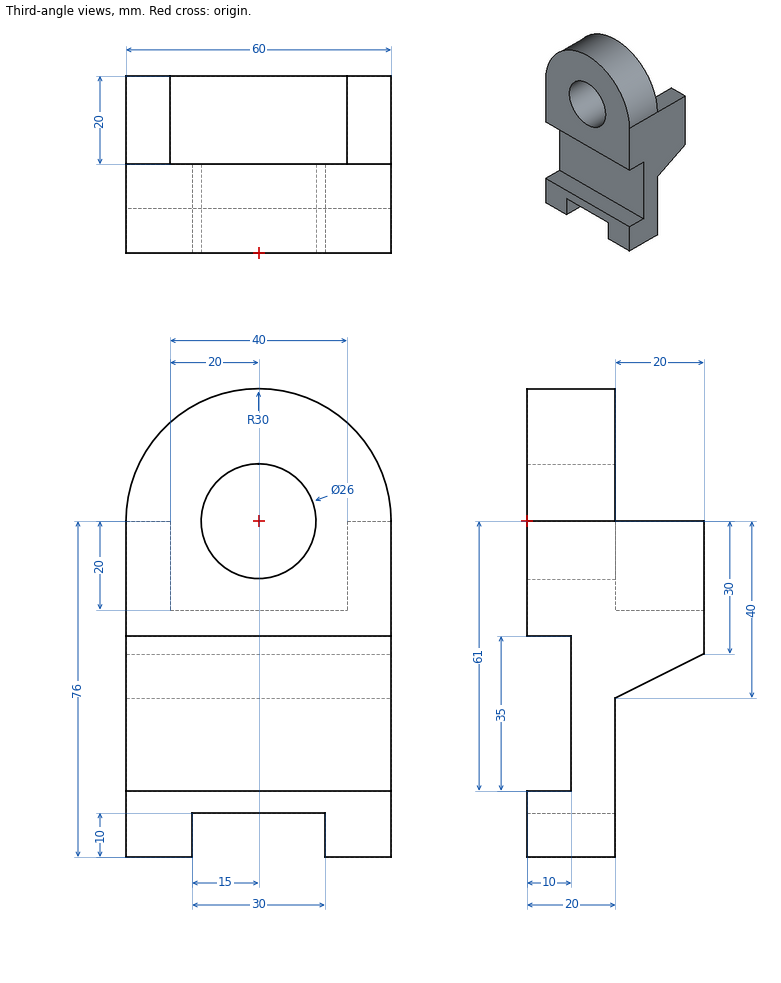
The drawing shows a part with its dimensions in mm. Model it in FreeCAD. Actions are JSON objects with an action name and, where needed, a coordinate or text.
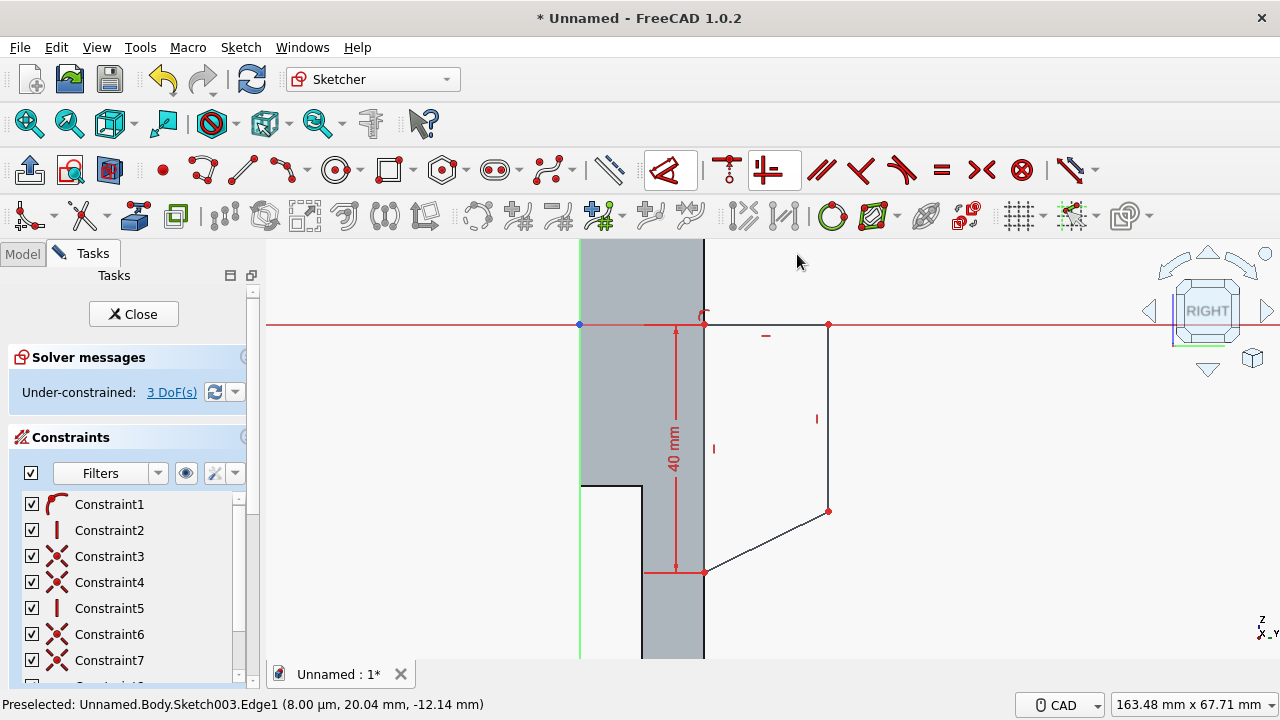
{"action": "left_click", "coordinate": [828, 456]}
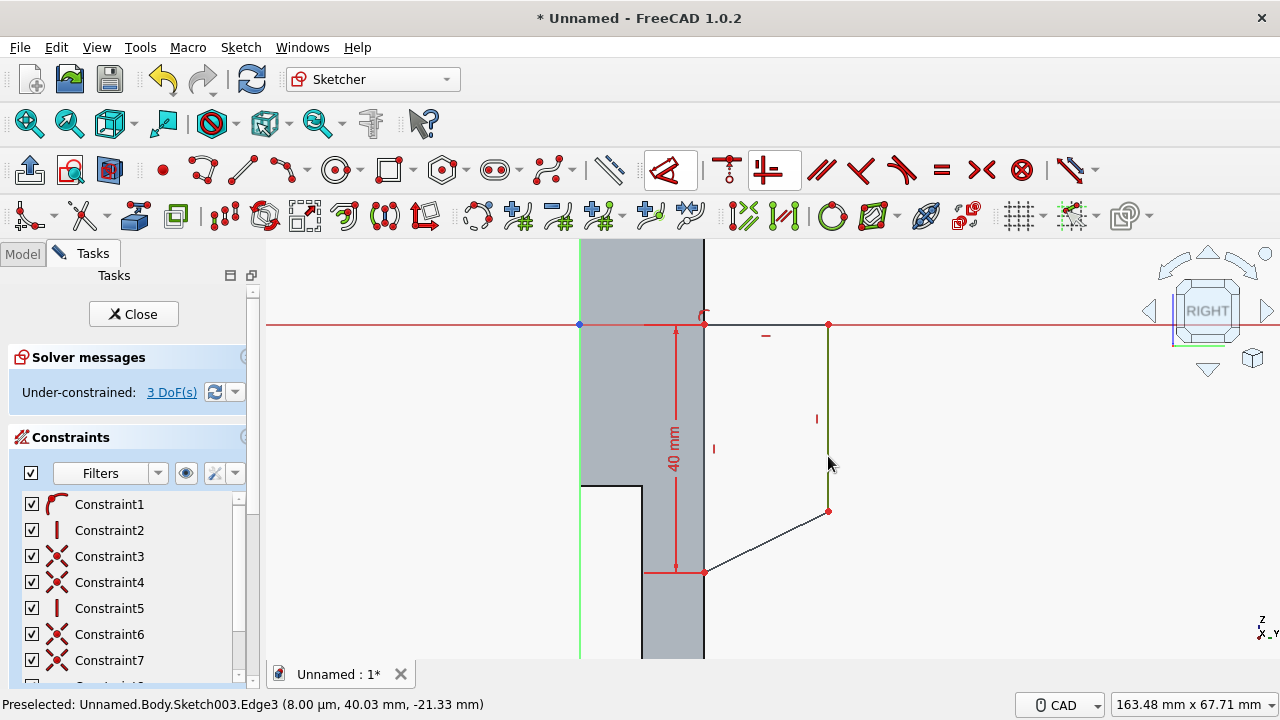
{"action": "key", "text": "i"}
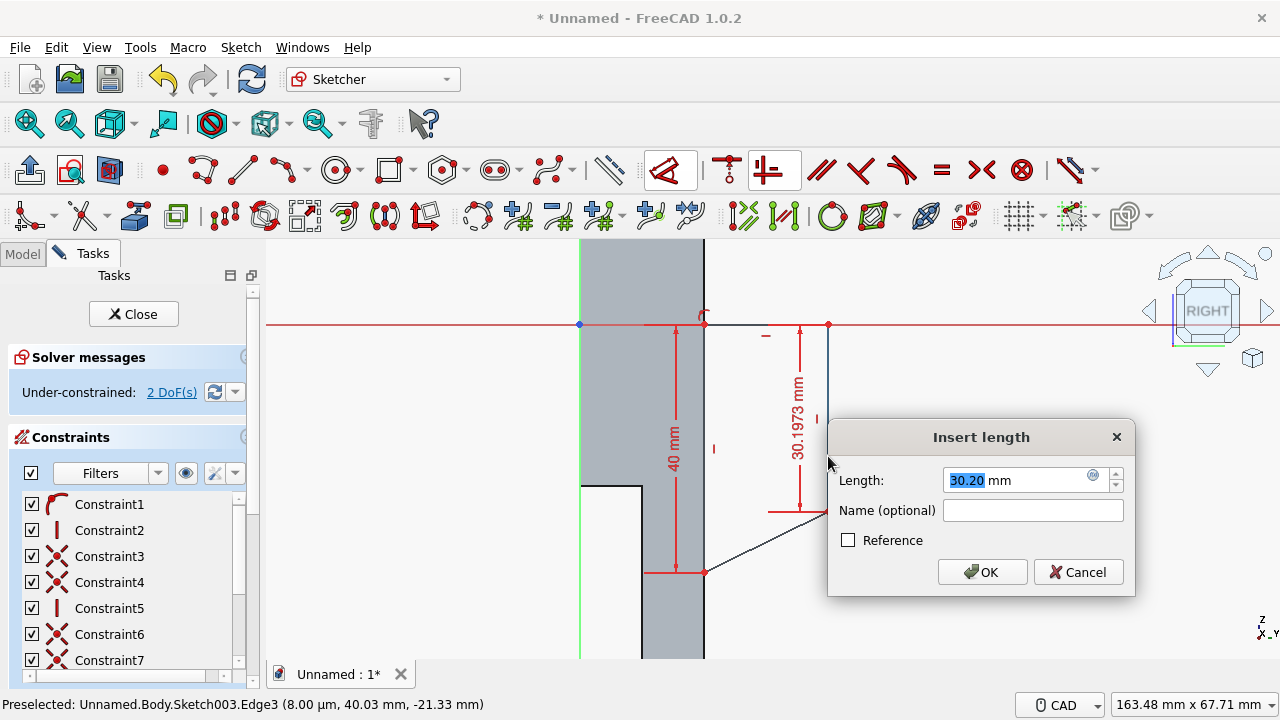
{"action": "type", "text": "30"}
{"action": "key", "text": "Return"}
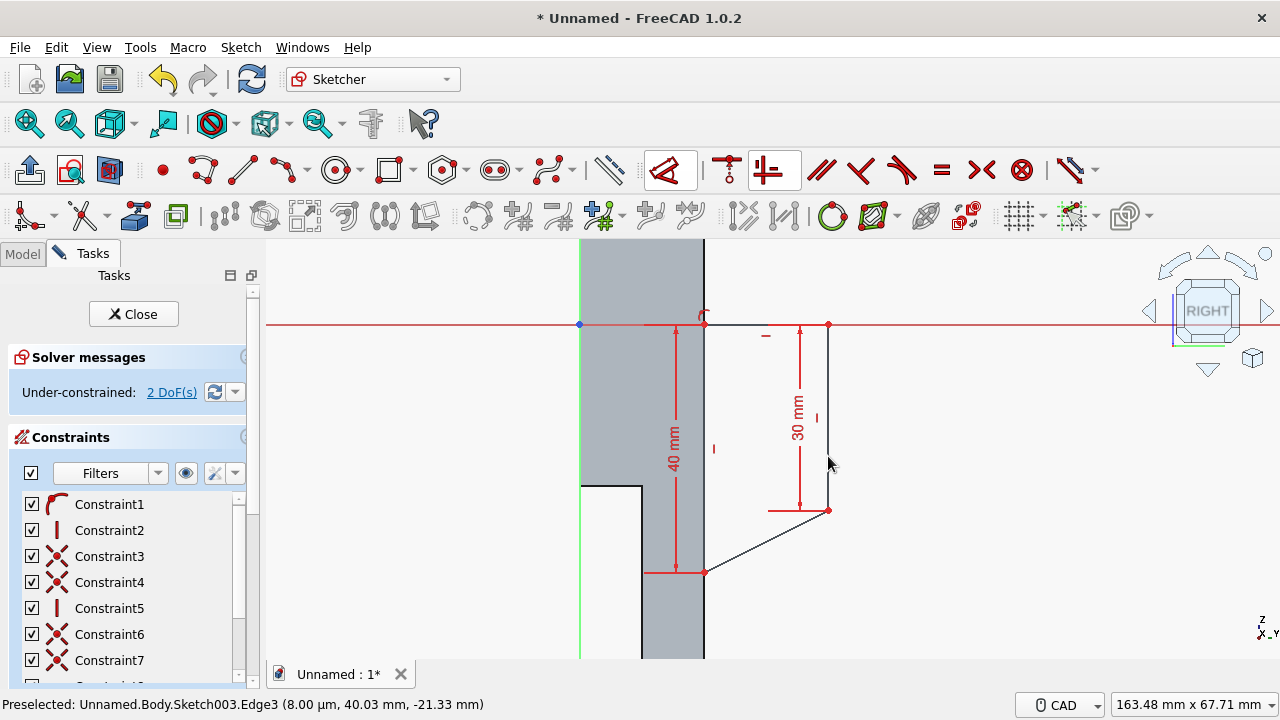
{"action": "left_click", "coordinate": [791, 325]}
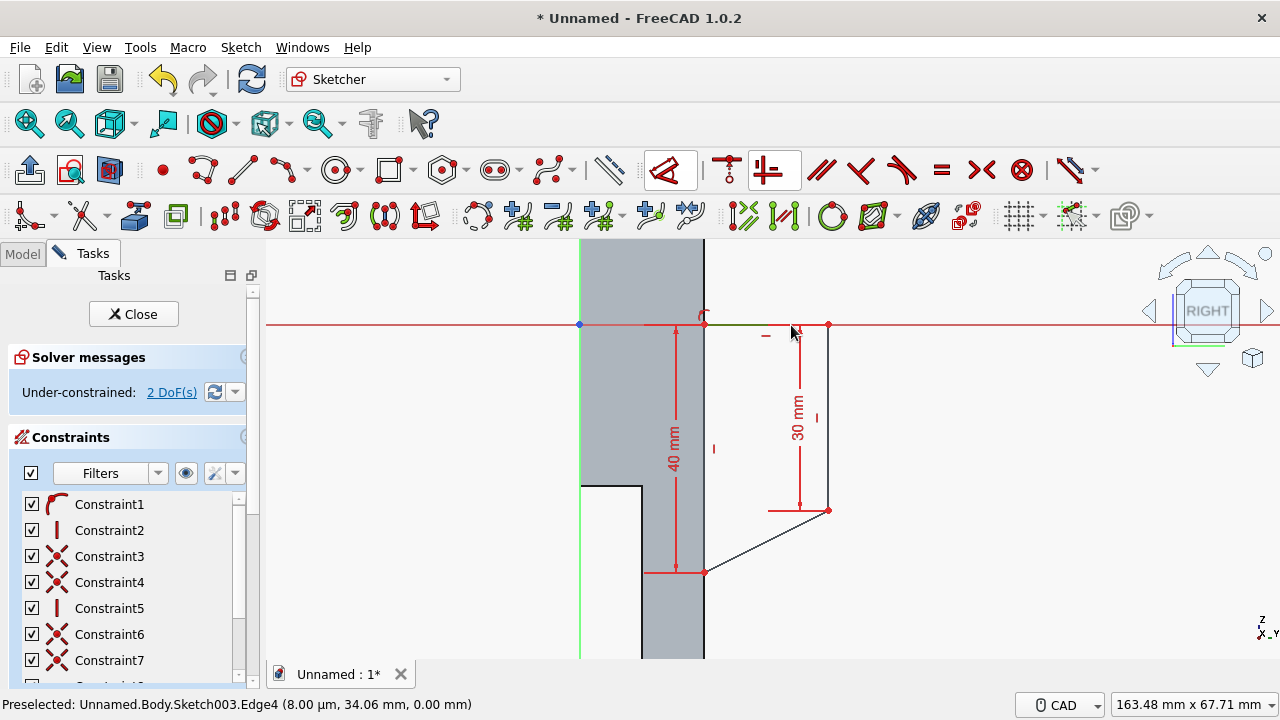
{"action": "left_click", "coordinate": [692, 170]}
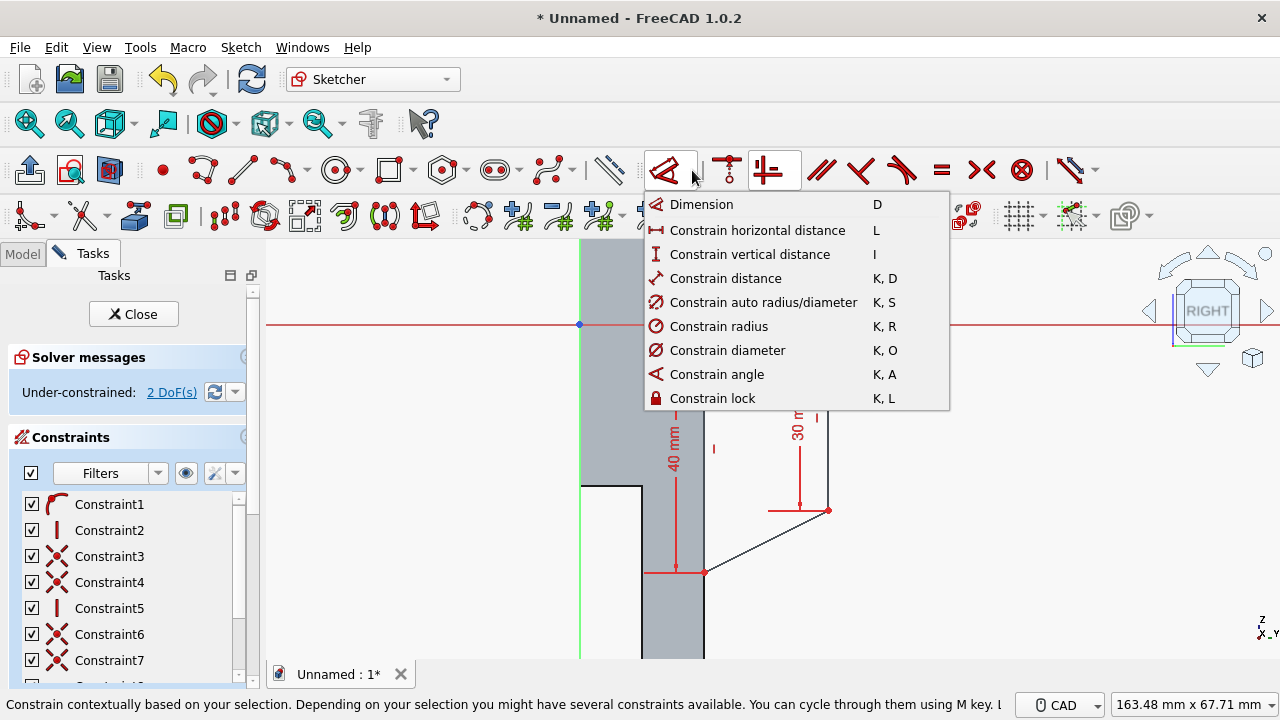
{"action": "left_click", "coordinate": [797, 230]}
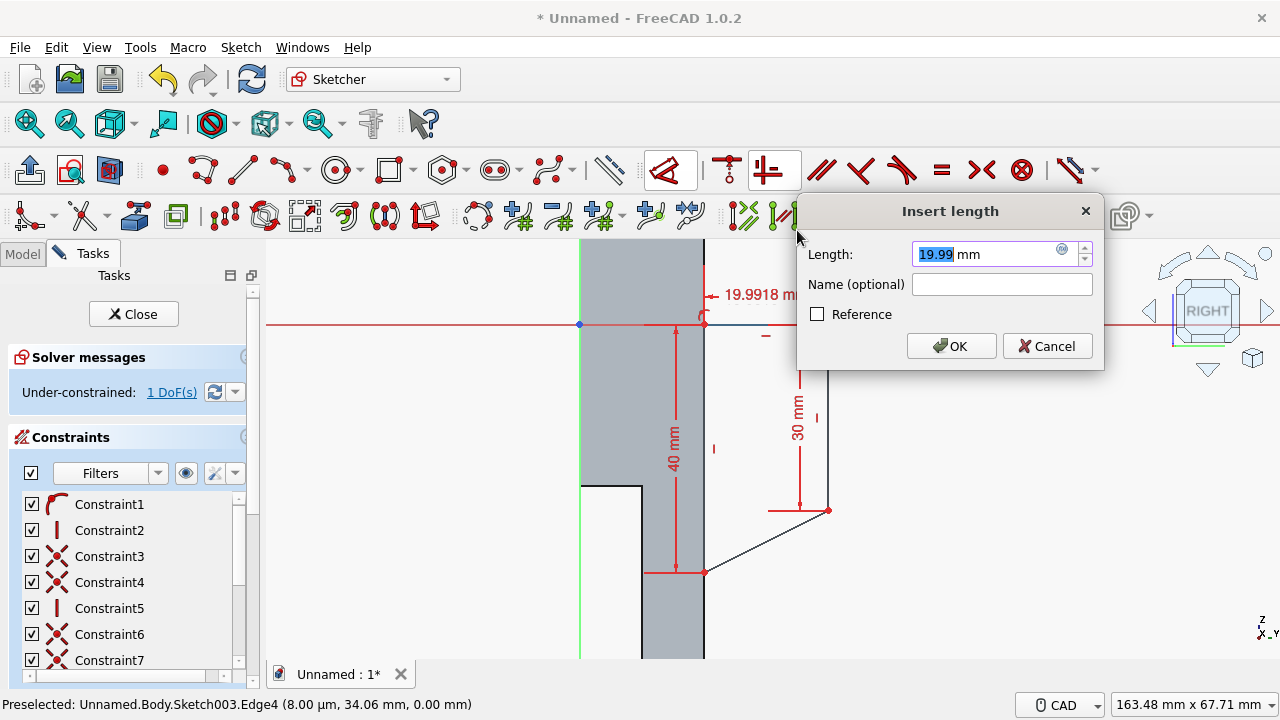
{"action": "type", "text": "20"}
{"action": "key", "text": "Return"}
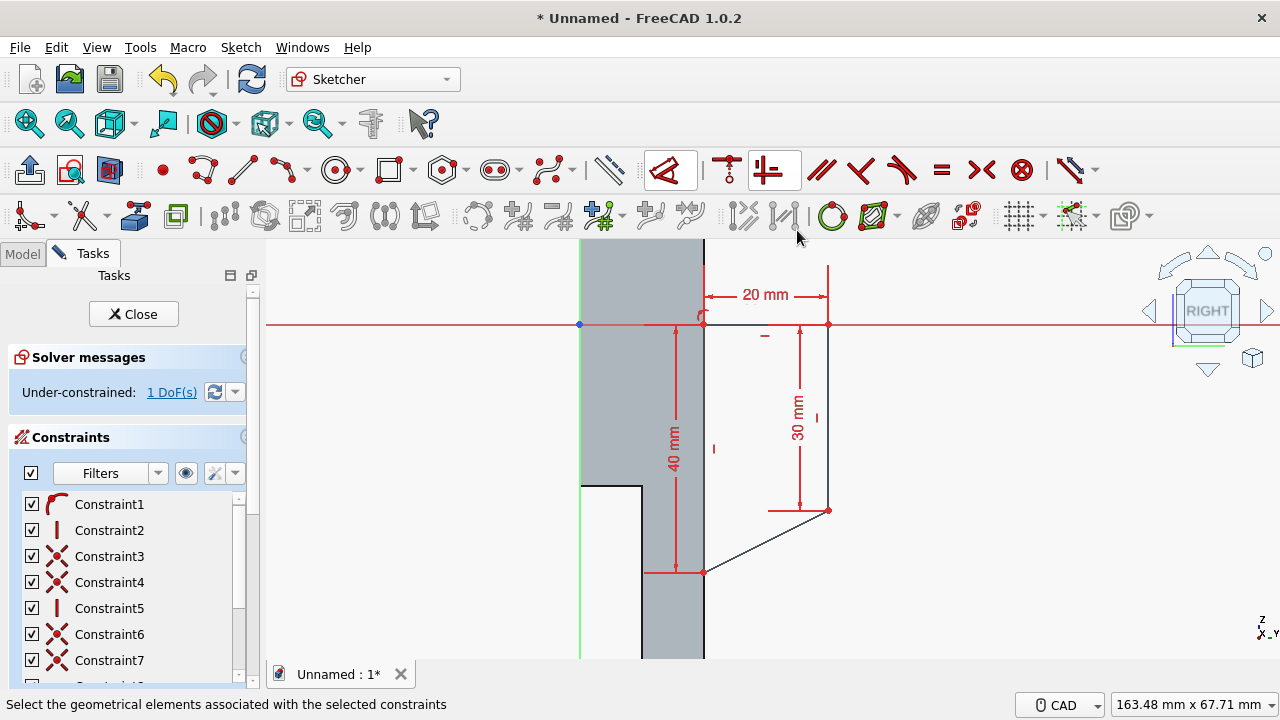
{"action": "left_click", "coordinate": [704, 325]}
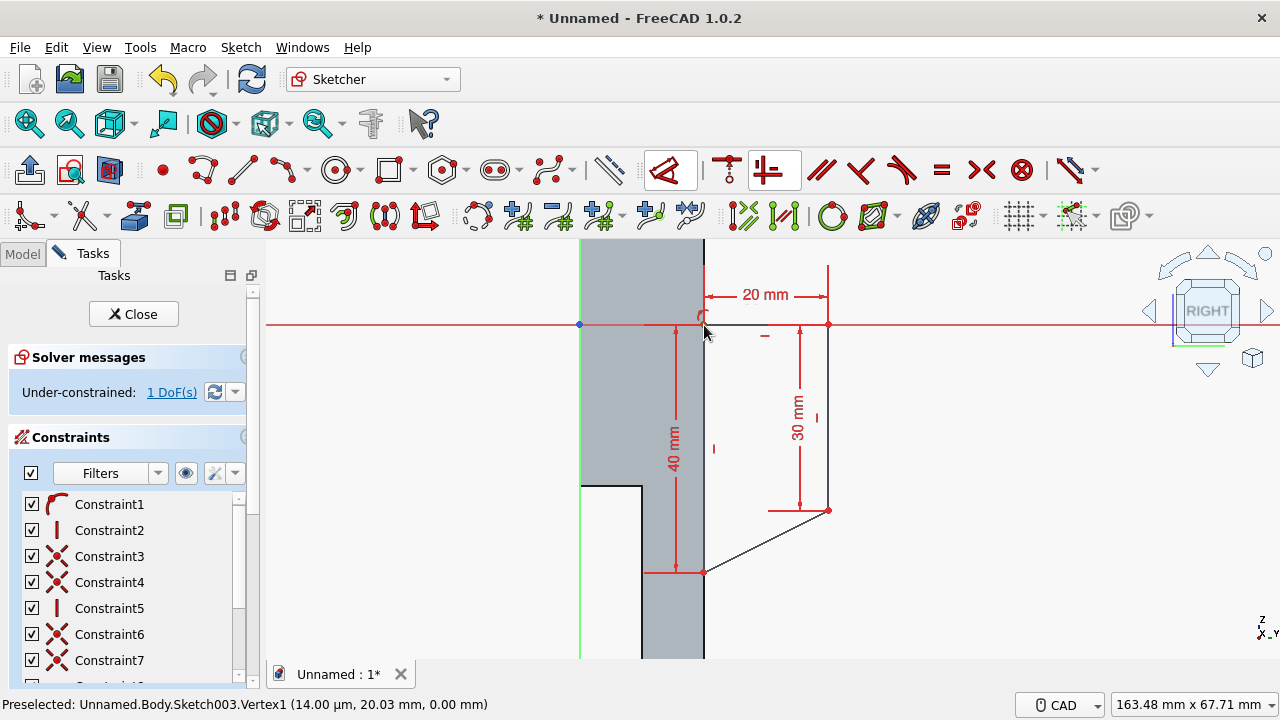
{"action": "key", "text": "l"}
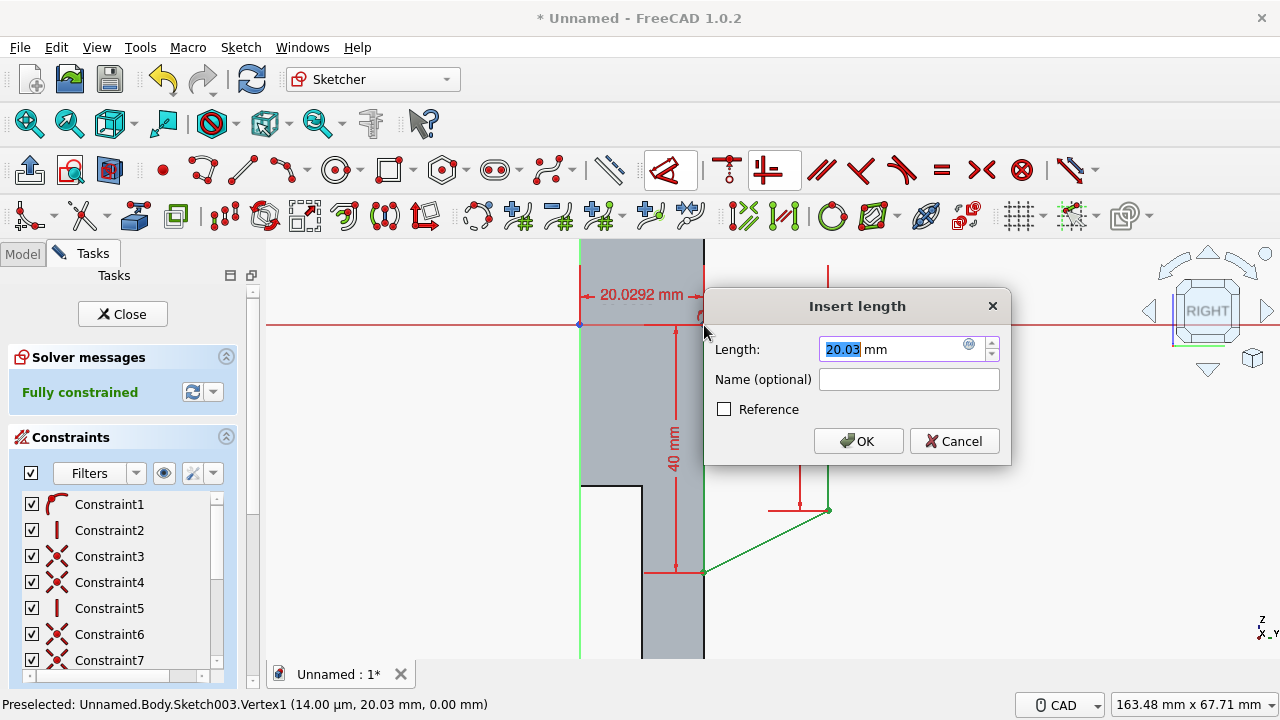
{"action": "type", "text": "20"}
{"action": "key", "text": "Return"}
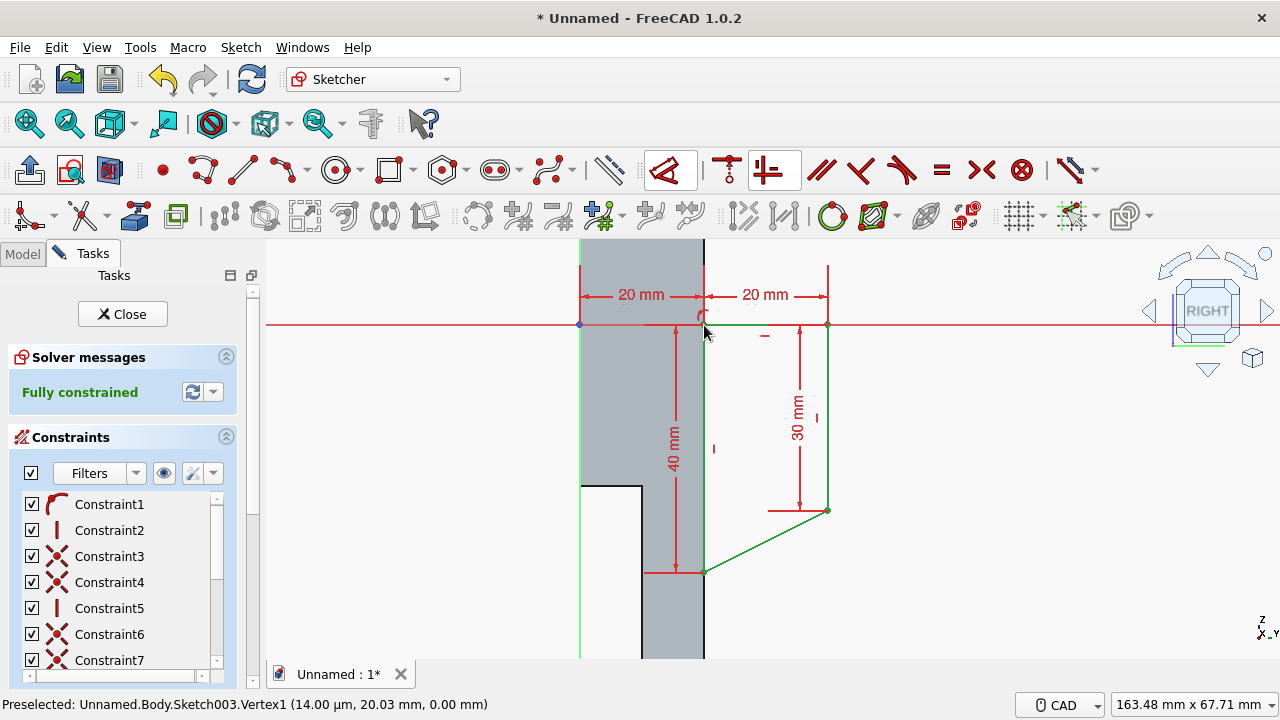
{"action": "left_click", "coordinate": [123, 314]}